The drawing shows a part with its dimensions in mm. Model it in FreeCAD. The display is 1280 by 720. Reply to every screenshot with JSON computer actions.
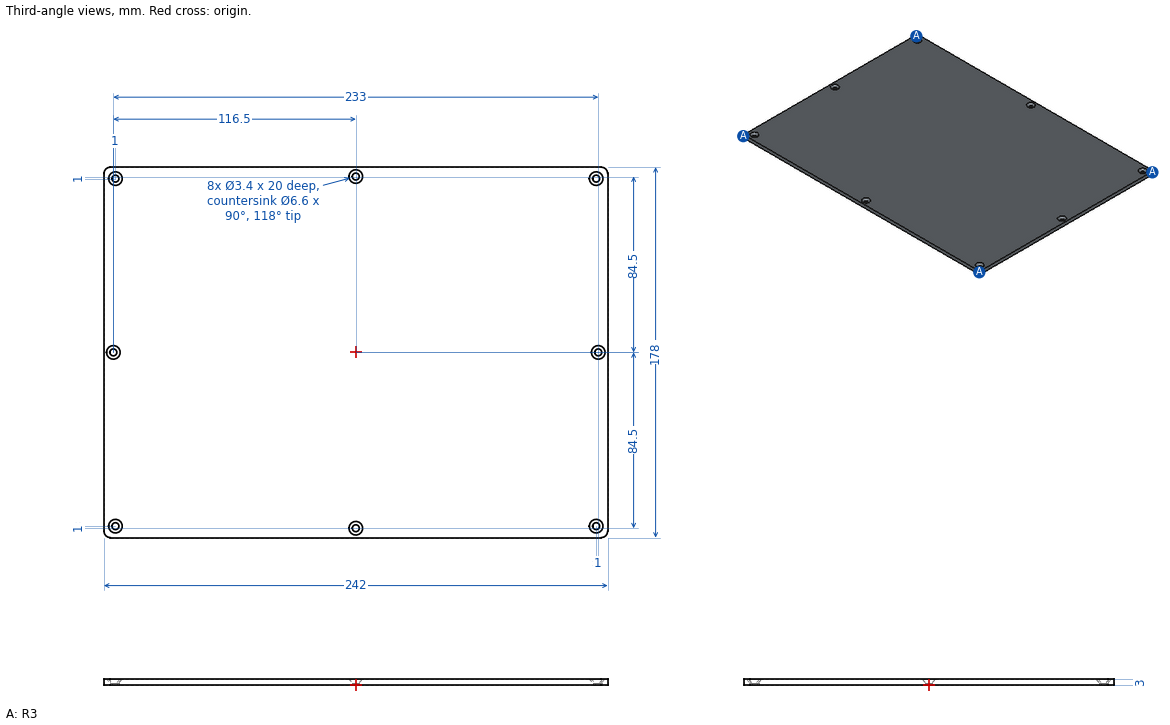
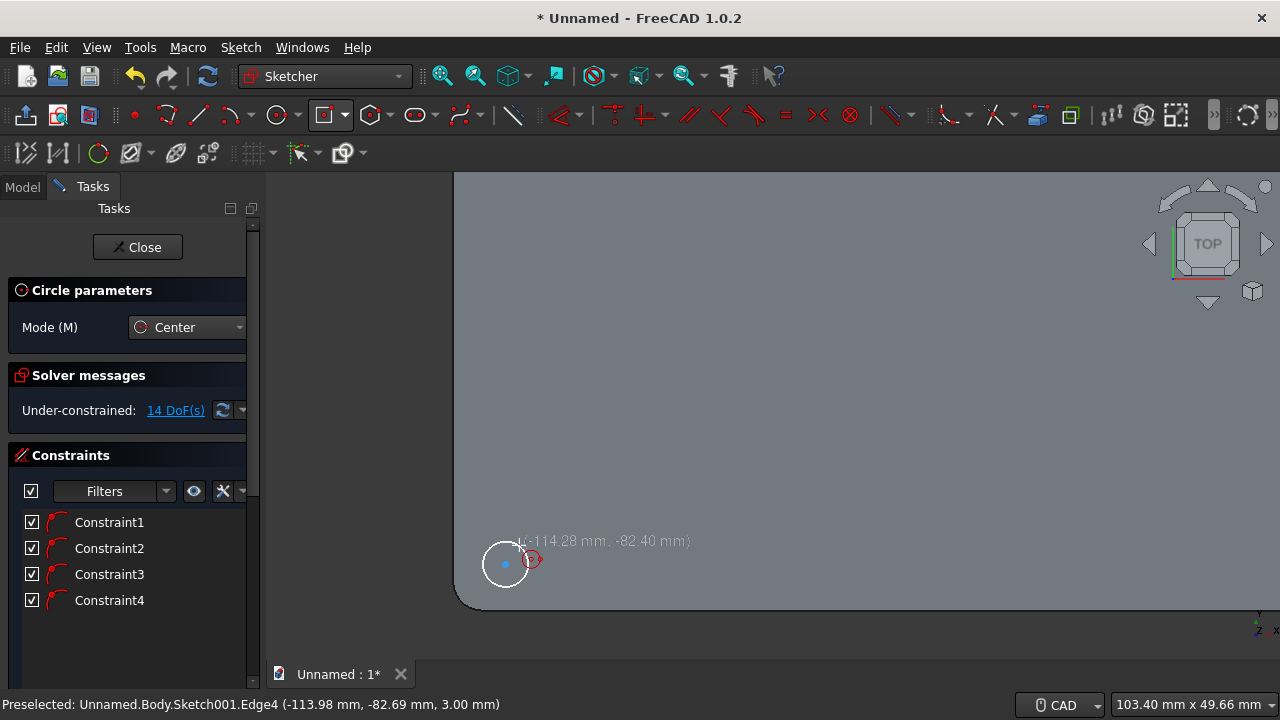
{"action": "scroll", "coordinate": [519, 550], "scroll_direction": "down", "scroll_amount": 9}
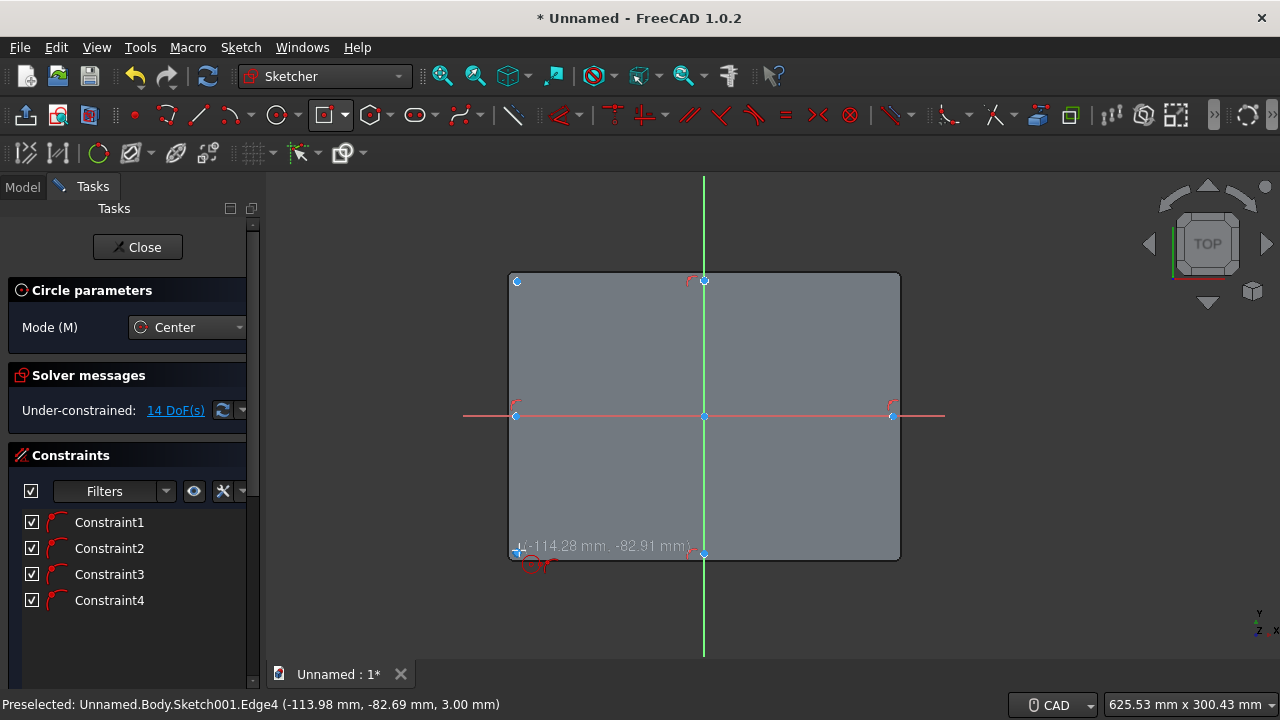
{"action": "scroll", "coordinate": [892, 552], "scroll_direction": "up", "scroll_amount": 11}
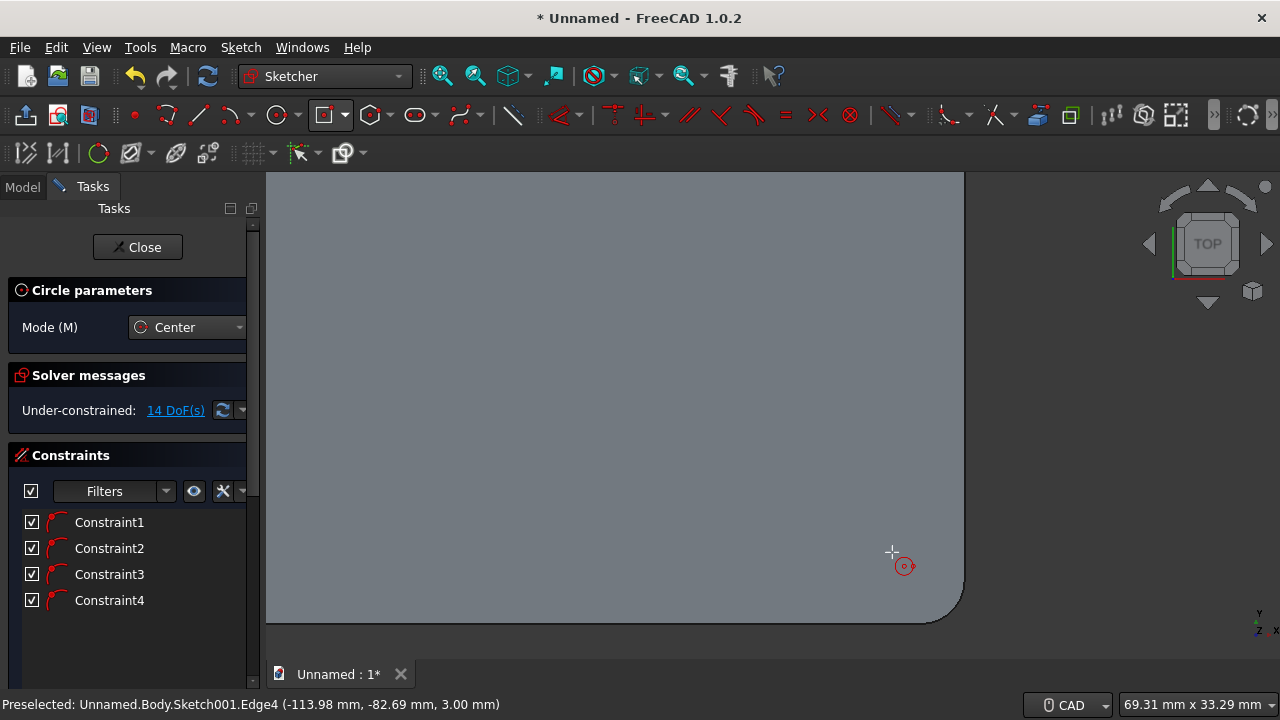
{"action": "scroll", "coordinate": [893, 552], "scroll_direction": "down", "scroll_amount": 11}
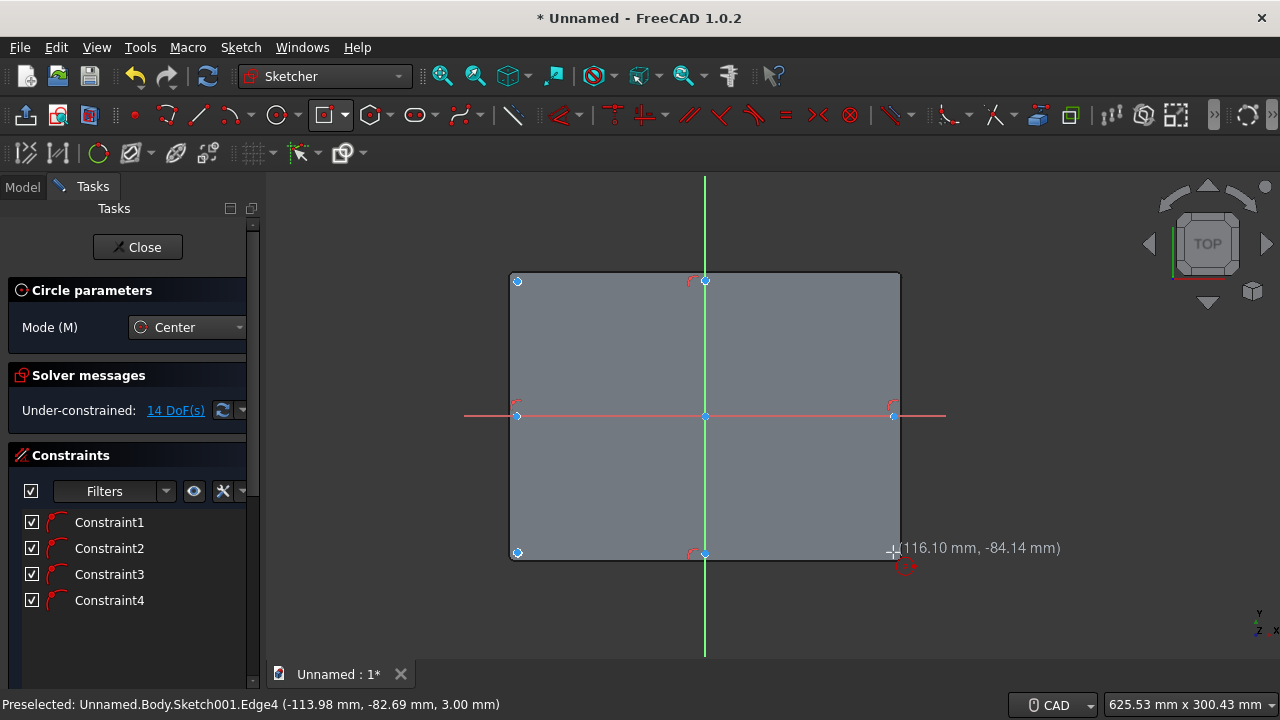
{"action": "left_click", "coordinate": [893, 552]}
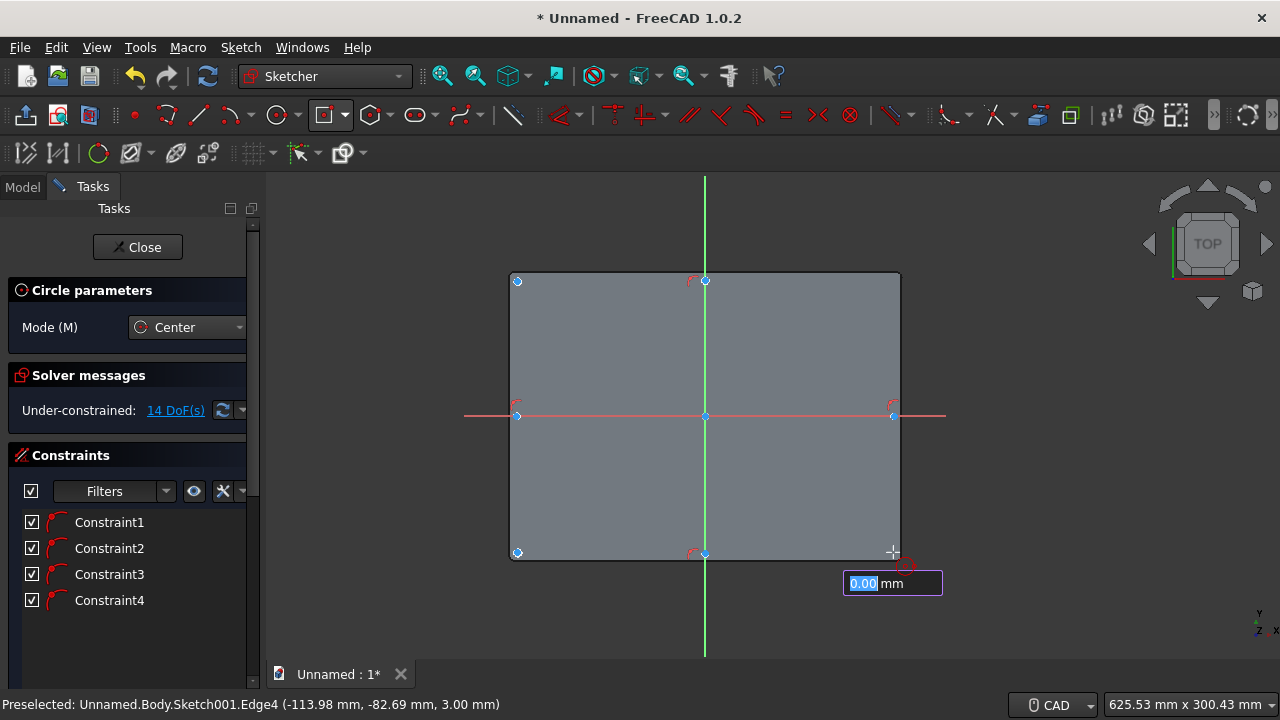
{"action": "scroll", "coordinate": [895, 550], "scroll_direction": "up", "scroll_amount": 9}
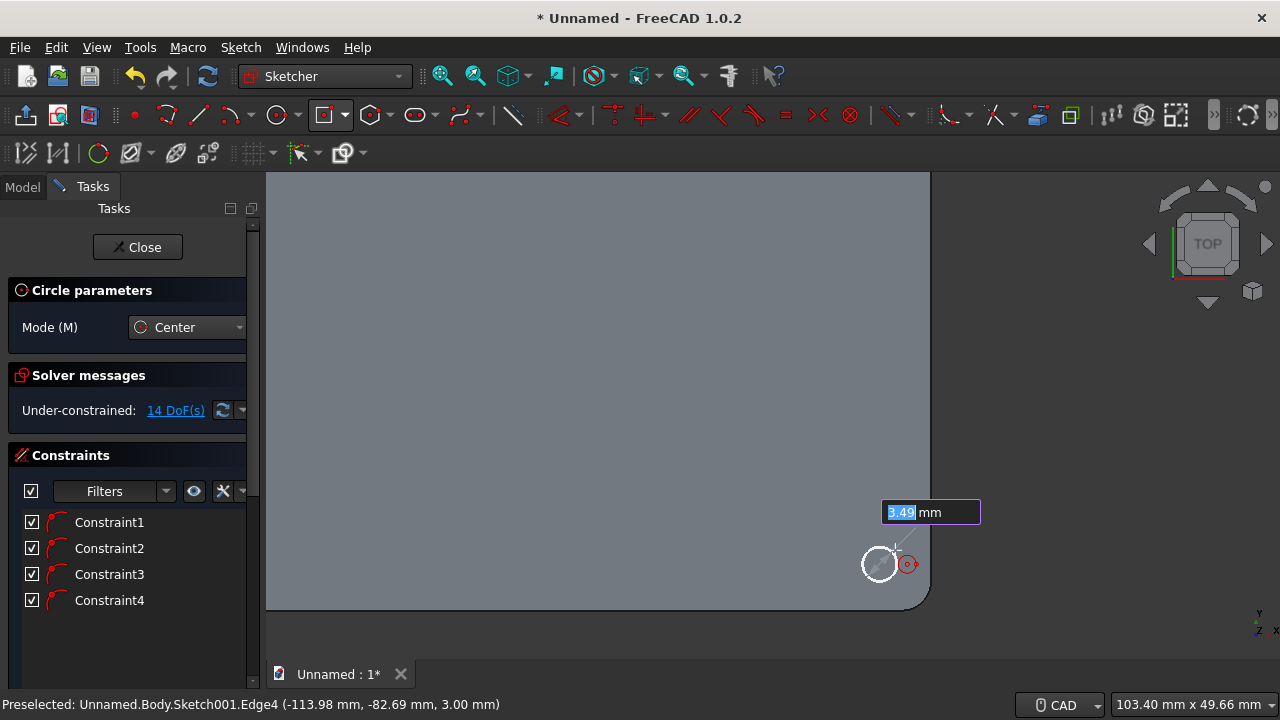
{"action": "left_click", "coordinate": [889, 545]}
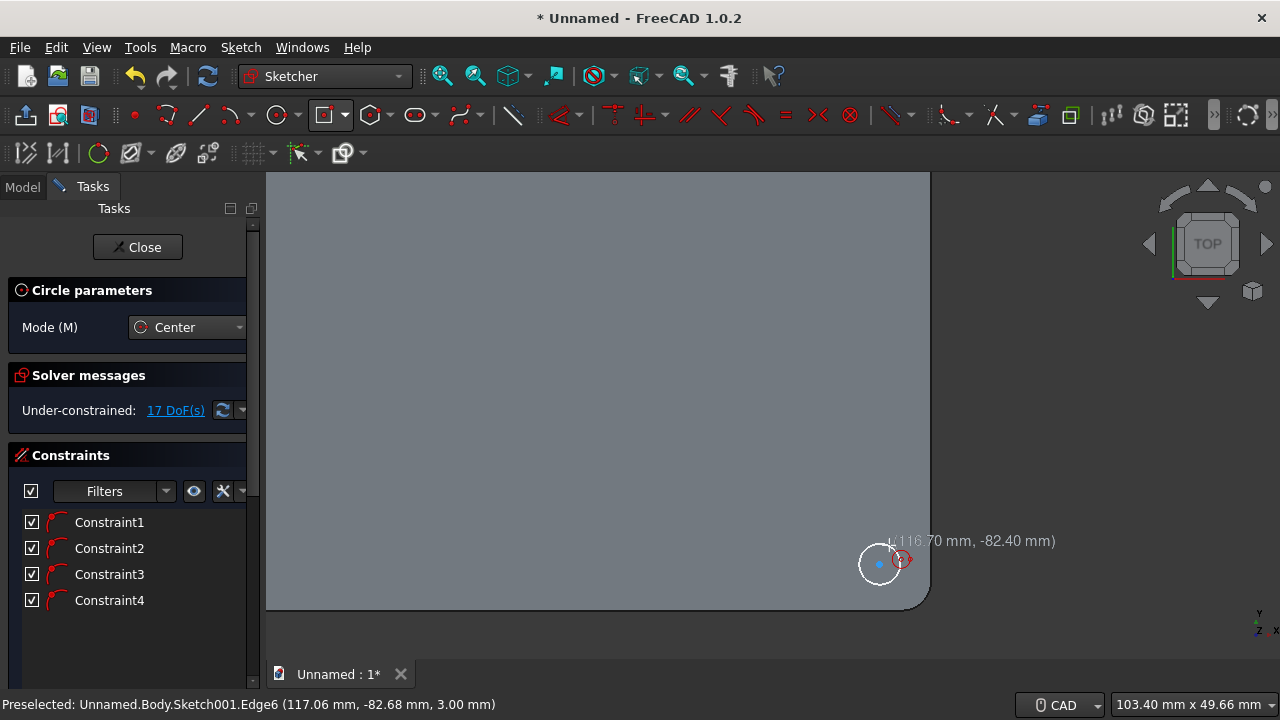
{"action": "scroll", "coordinate": [895, 550], "scroll_direction": "down", "scroll_amount": 9}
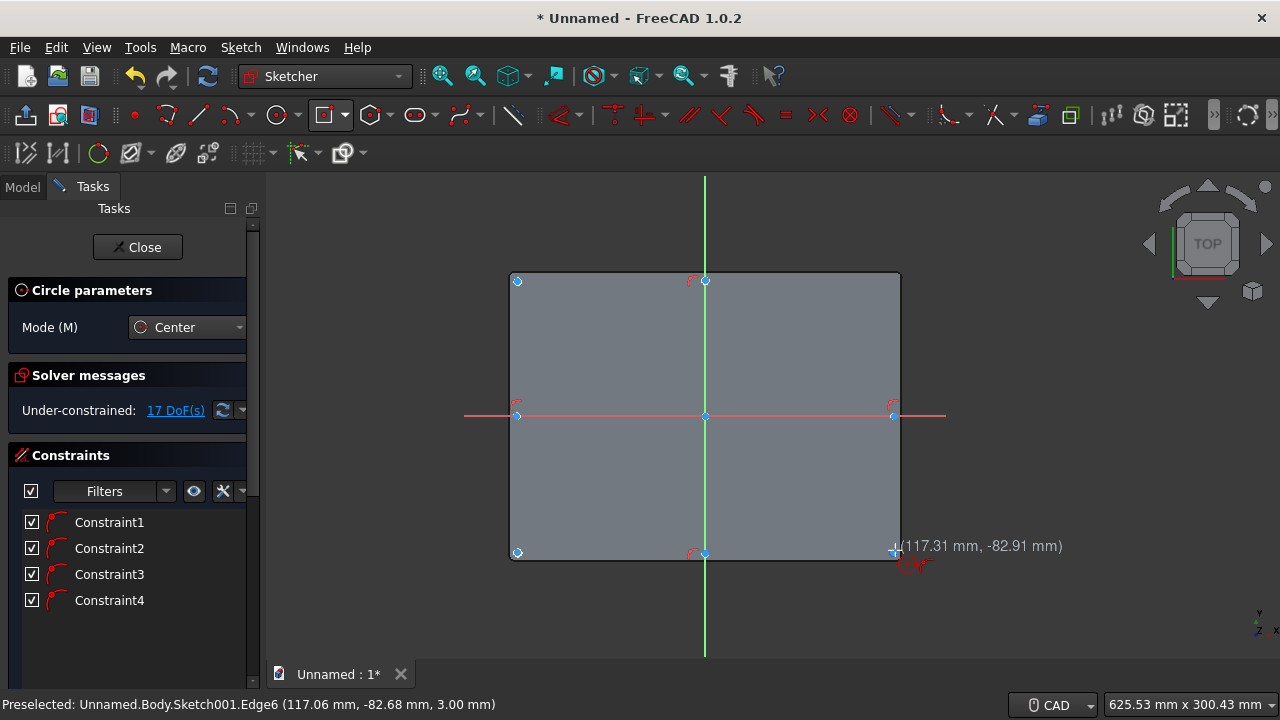
{"action": "scroll", "coordinate": [893, 281], "scroll_direction": "up", "scroll_amount": 11}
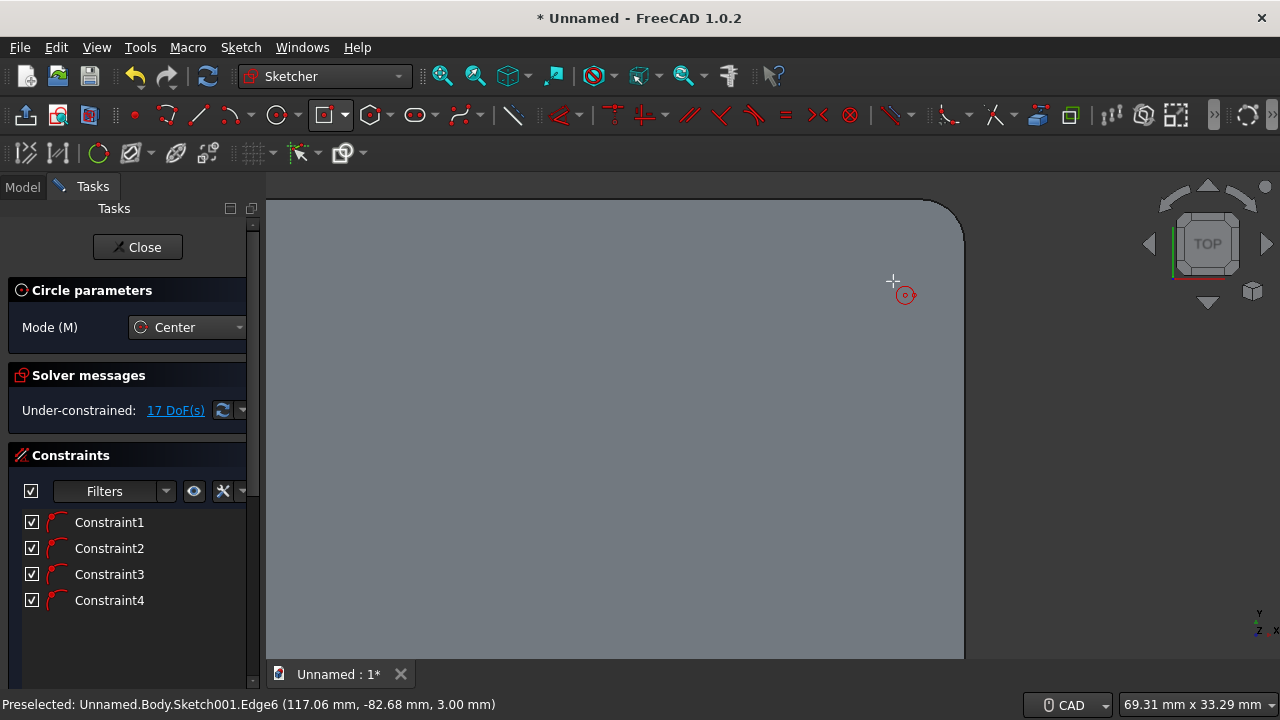
{"action": "scroll", "coordinate": [893, 280], "scroll_direction": "down", "scroll_amount": 11}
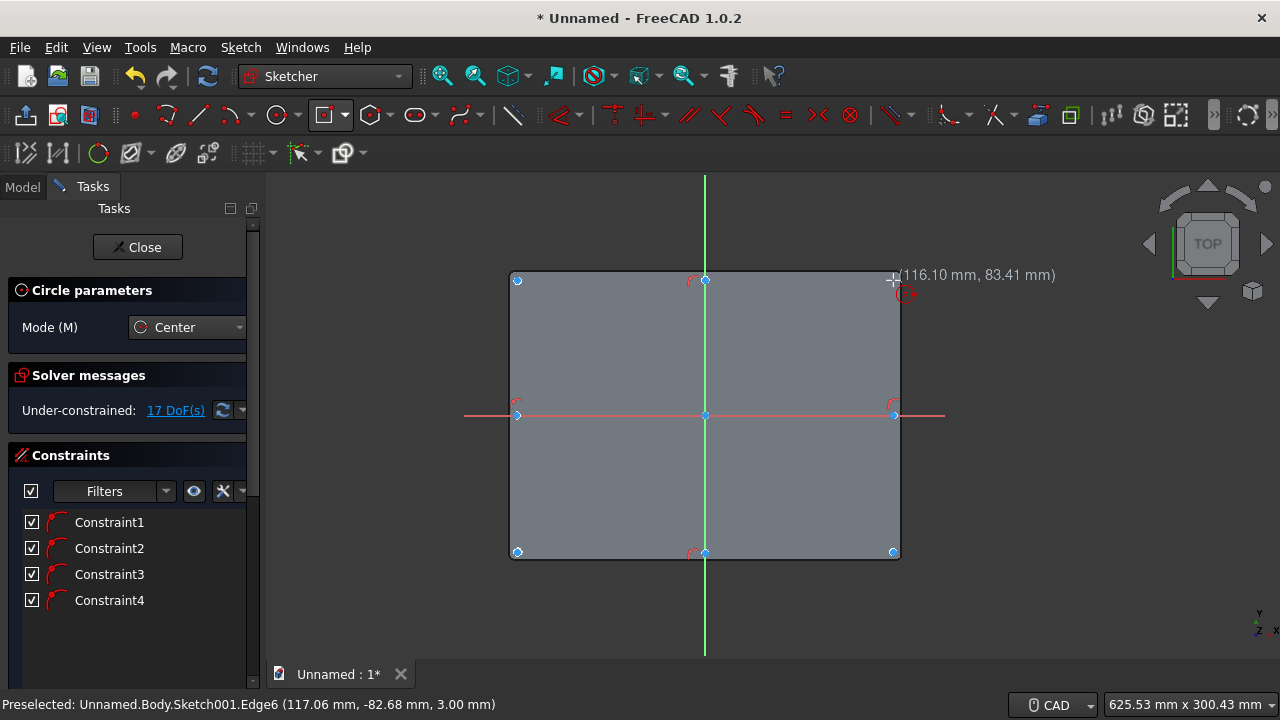
{"action": "left_click", "coordinate": [893, 280]}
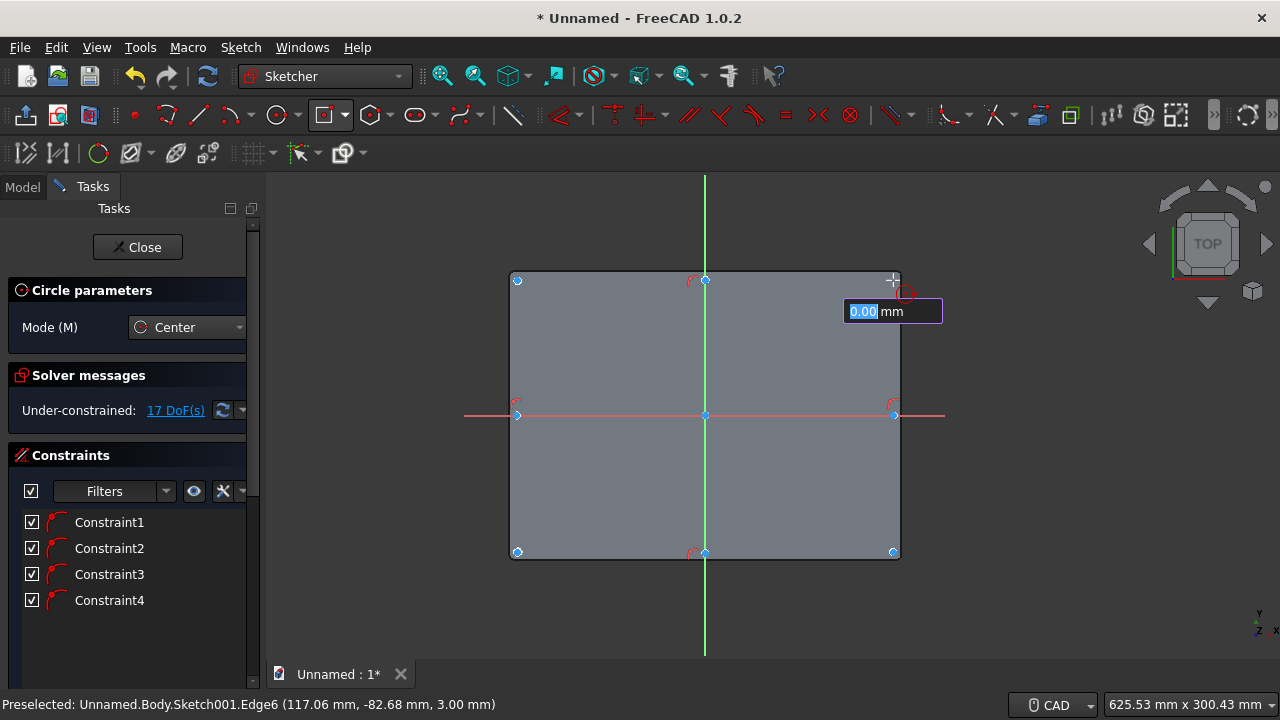
{"action": "scroll", "coordinate": [895, 278], "scroll_direction": "up", "scroll_amount": 9}